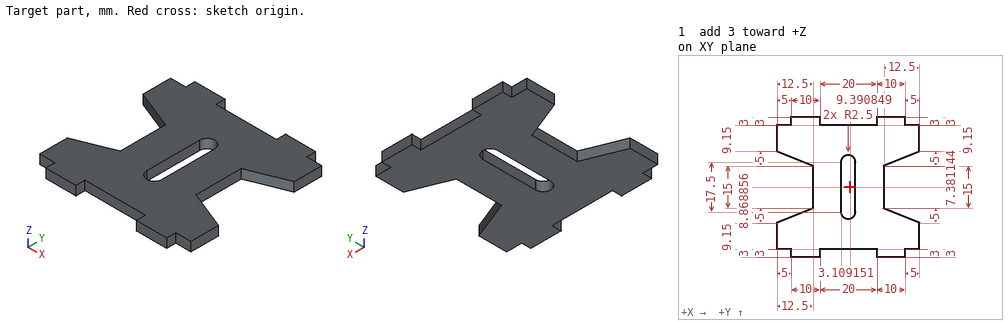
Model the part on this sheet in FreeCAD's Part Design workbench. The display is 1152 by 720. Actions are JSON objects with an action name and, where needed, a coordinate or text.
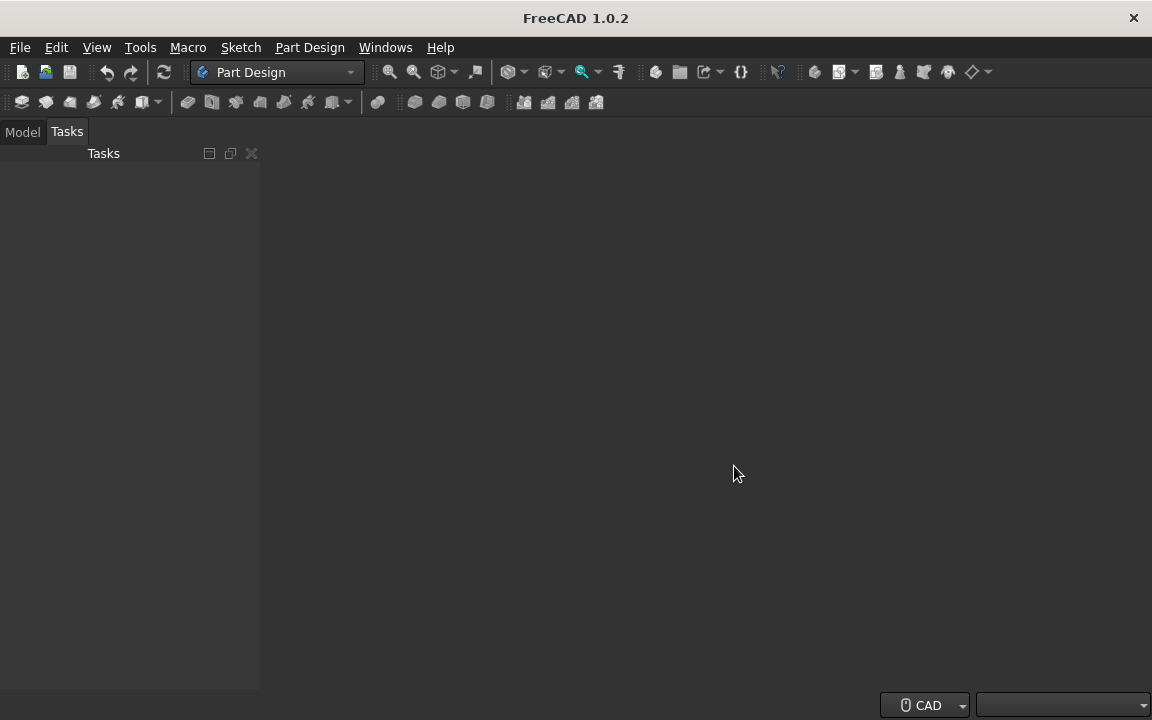
{"action": "left_click", "coordinate": [22, 72]}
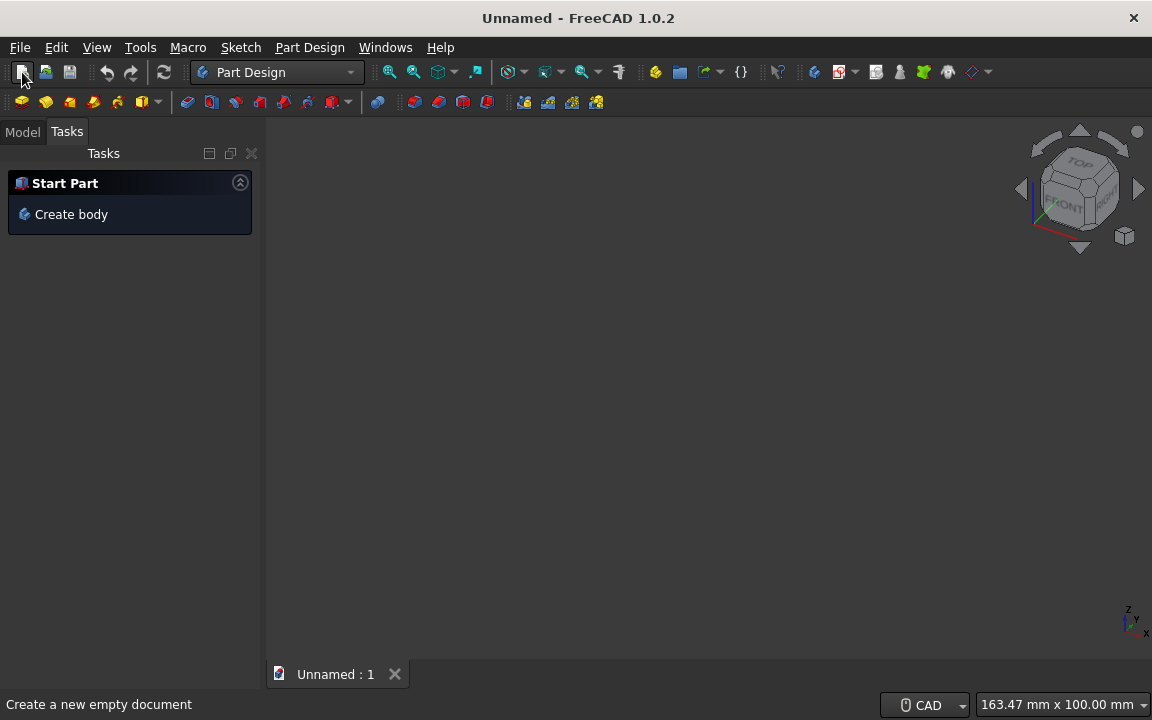
{"action": "left_click", "coordinate": [840, 72]}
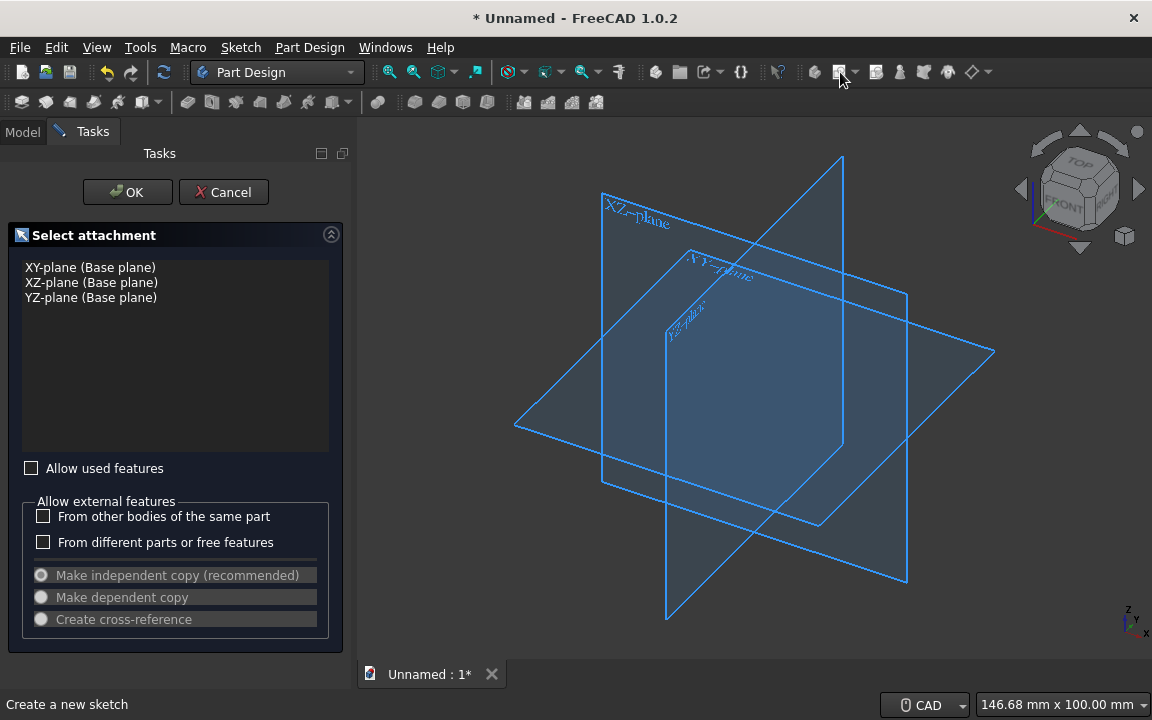
{"action": "left_click", "coordinate": [82, 268]}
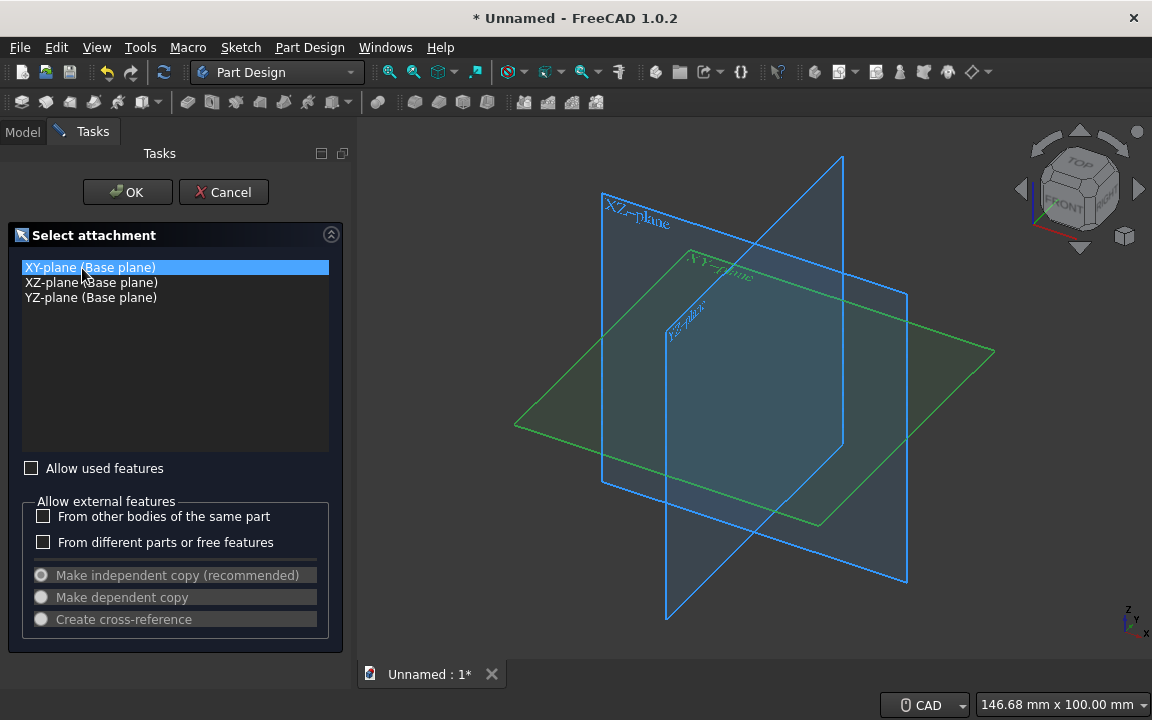
{"action": "left_click", "coordinate": [128, 192]}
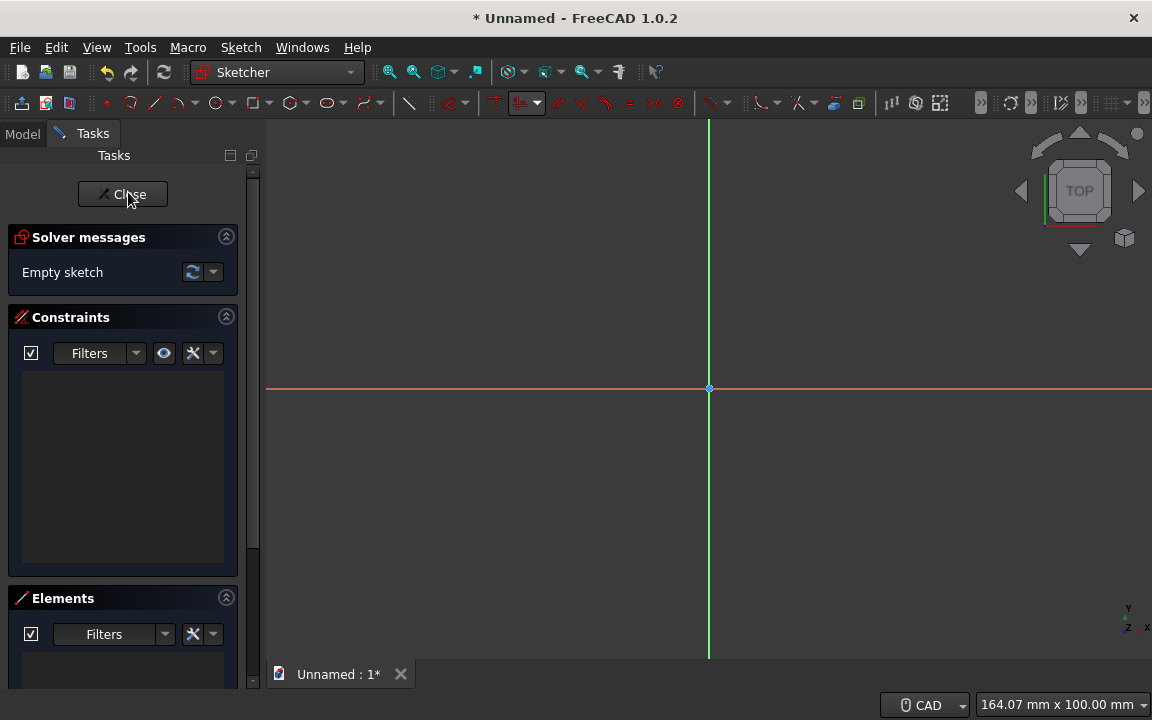
{"action": "left_click", "coordinate": [132, 104]}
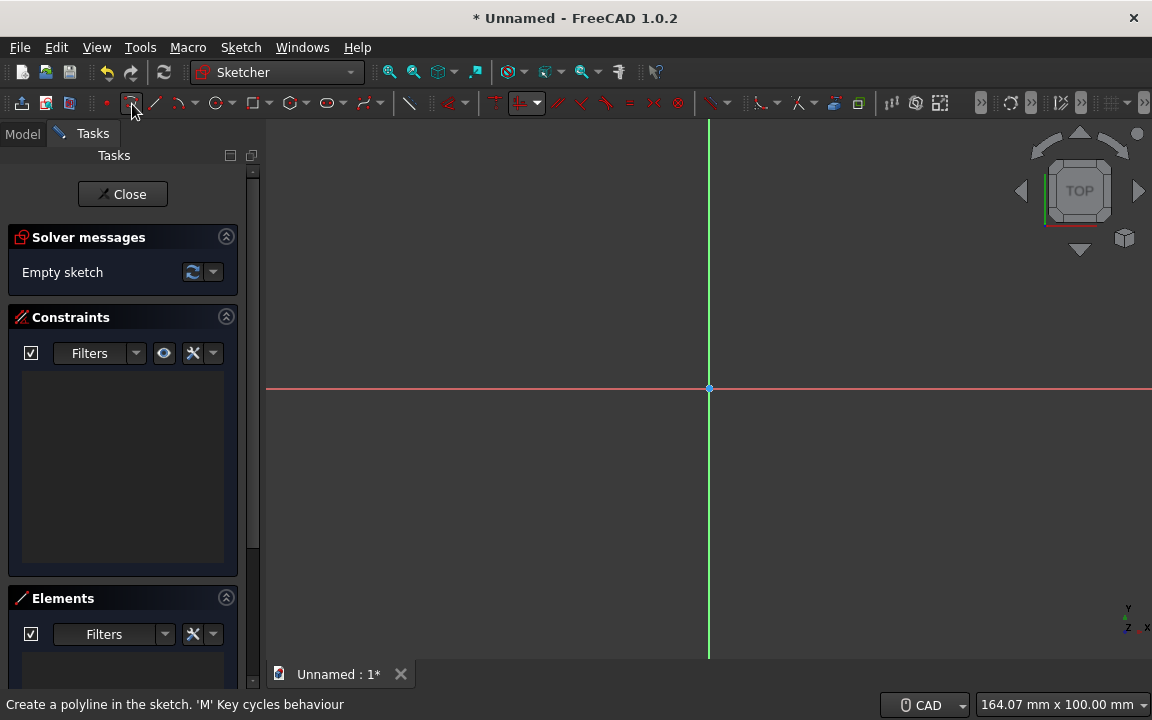
{"action": "left_click", "coordinate": [773, 349]}
{"action": "left_click", "coordinate": [841, 322]}
{"action": "left_click", "coordinate": [841, 273]}
{"action": "left_click", "coordinate": [814, 273]}
{"action": "left_click", "coordinate": [814, 257]}
{"action": "left_click", "coordinate": [760, 257]}
{"action": "left_click", "coordinate": [760, 273]}
{"action": "left_click", "coordinate": [652, 273]}
{"action": "left_click", "coordinate": [652, 257]}
{"action": "left_click", "coordinate": [598, 257]}
{"action": "left_click", "coordinate": [598, 273]}
{"action": "left_click", "coordinate": [571, 273]}
{"action": "left_click", "coordinate": [571, 322]}
{"action": "left_click", "coordinate": [638, 349]}
{"action": "left_click", "coordinate": [638, 430]}
{"action": "left_click", "coordinate": [571, 457]}
{"action": "left_click", "coordinate": [571, 507]}
{"action": "left_click", "coordinate": [598, 507]}
{"action": "left_click", "coordinate": [598, 523]}
{"action": "left_click", "coordinate": [652, 523]}
{"action": "left_click", "coordinate": [652, 507]}
{"action": "left_click", "coordinate": [760, 507]}
{"action": "left_click", "coordinate": [760, 523]}
{"action": "left_click", "coordinate": [814, 523]}
{"action": "left_click", "coordinate": [814, 507]}
{"action": "left_click", "coordinate": [841, 507]}
{"action": "left_click", "coordinate": [841, 457]}
{"action": "left_click", "coordinate": [773, 430]}
{"action": "left_click", "coordinate": [773, 350]}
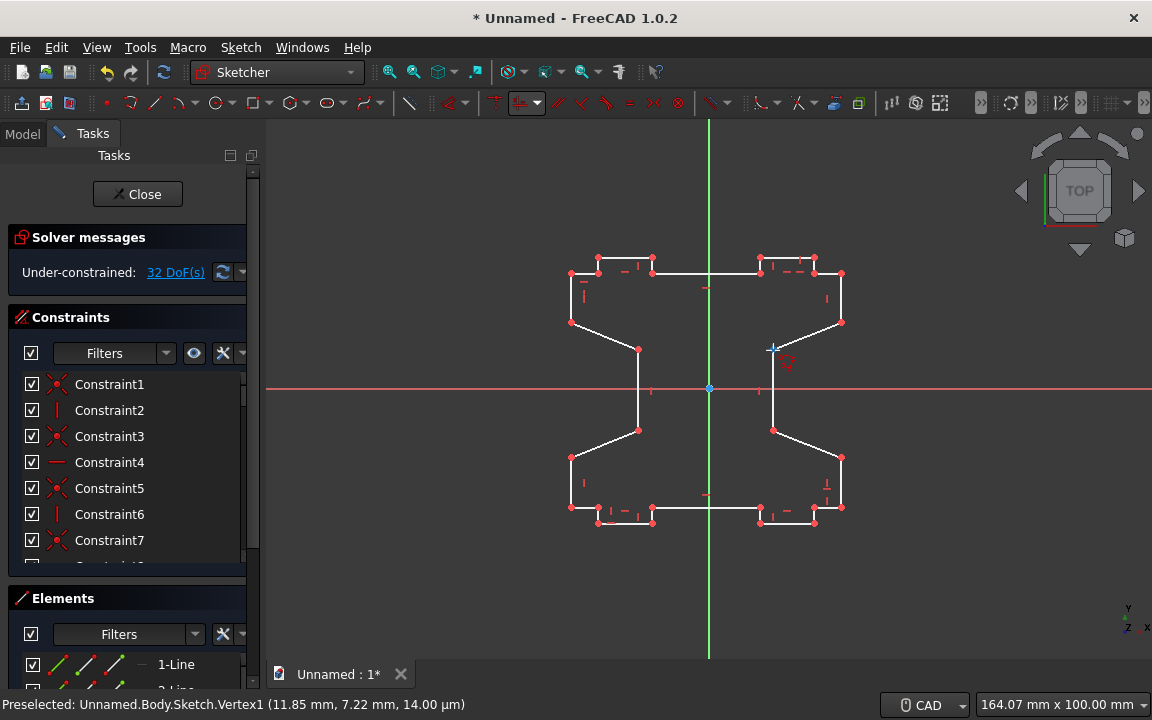
{"action": "left_click", "coordinate": [328, 104]}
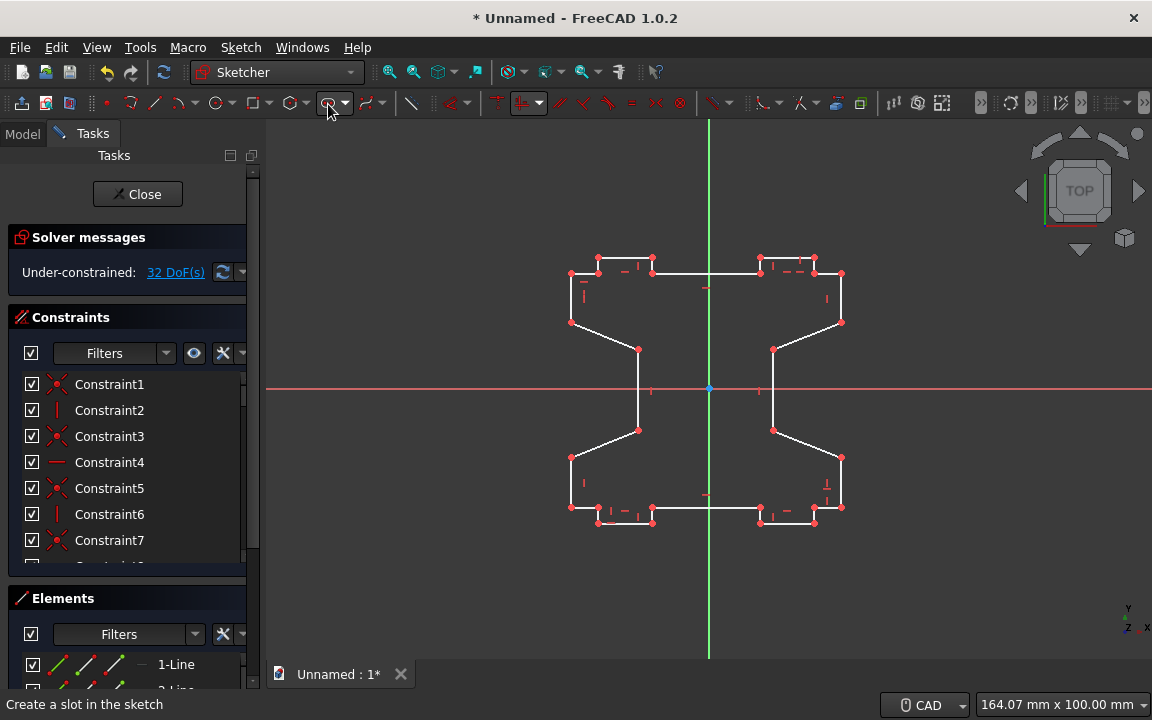
{"action": "scroll", "coordinate": [706, 437], "scroll_direction": "up", "scroll_amount": 8}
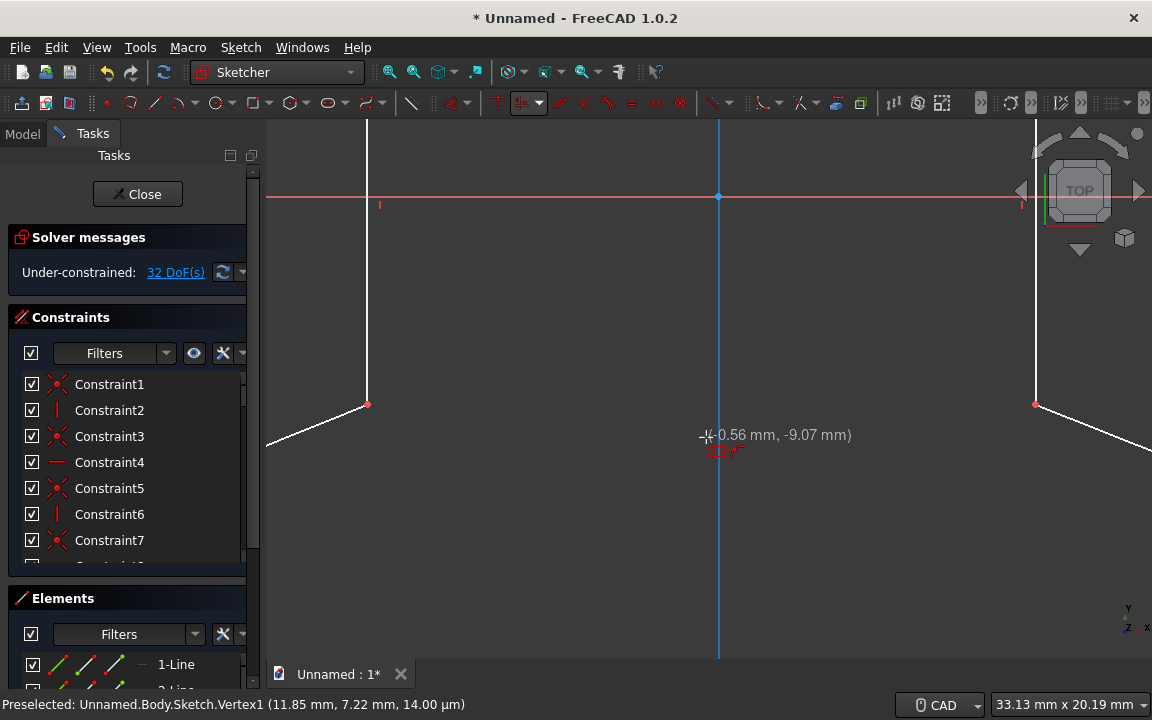
{"action": "left_click", "coordinate": [703, 434]}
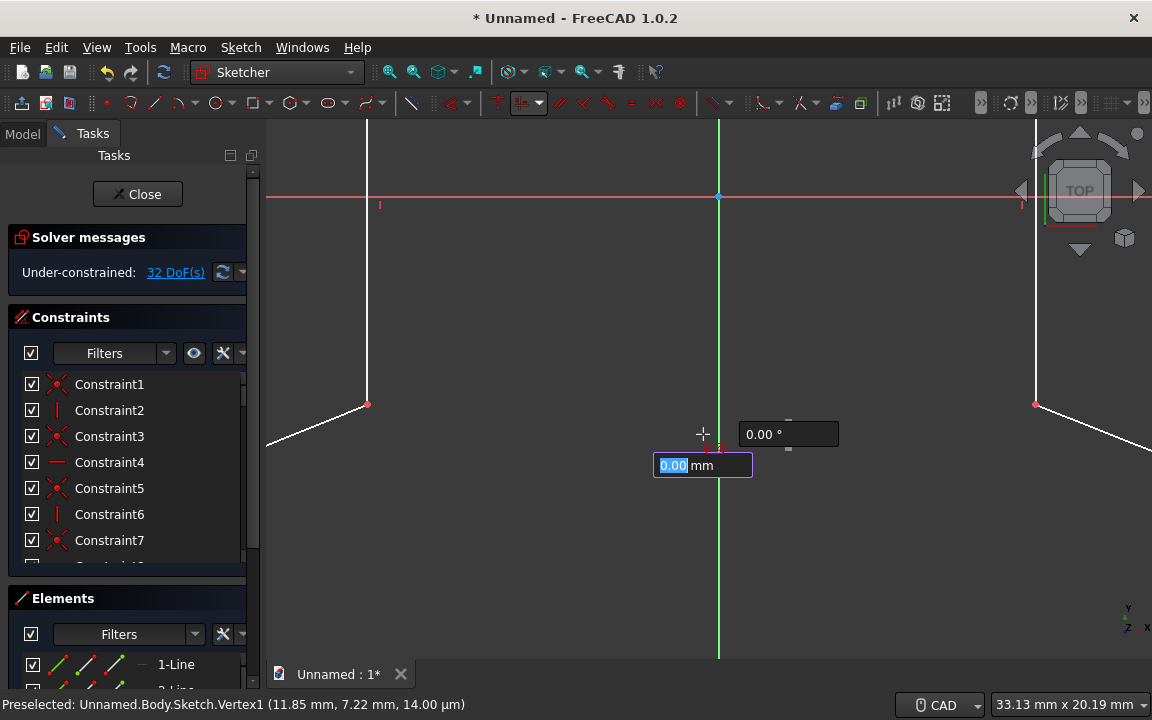
{"action": "scroll", "coordinate": [620, 451], "scroll_direction": "down", "scroll_amount": 7}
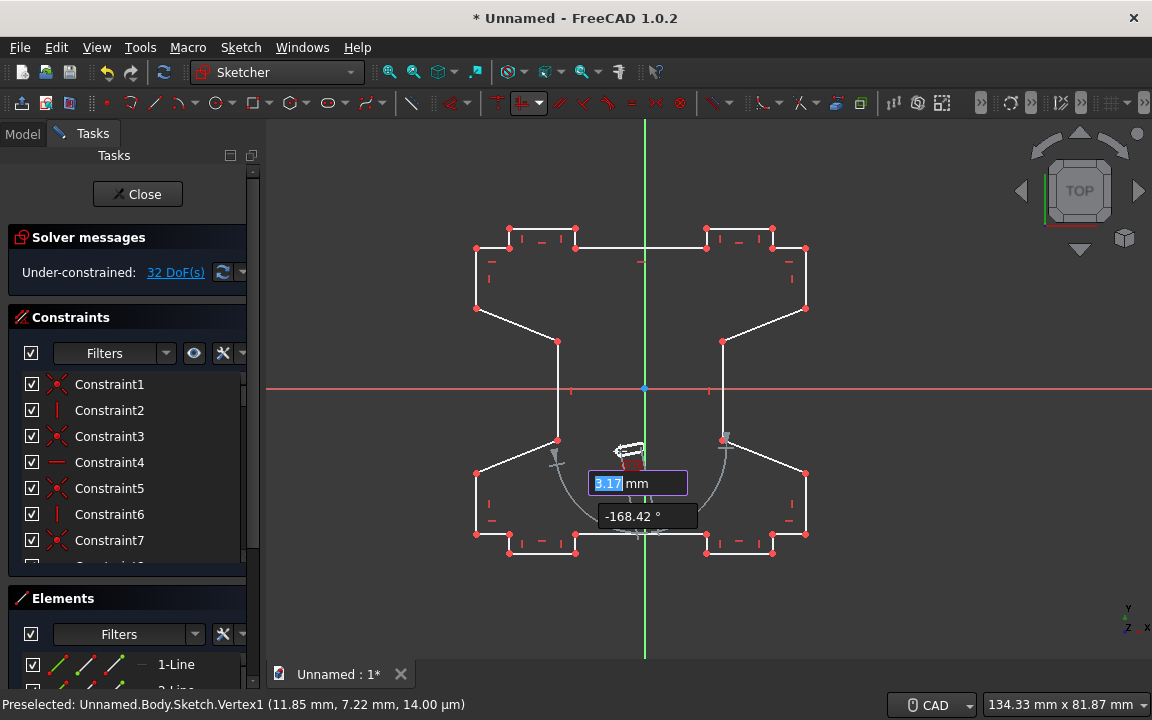
{"action": "scroll", "coordinate": [641, 332], "scroll_direction": "up", "scroll_amount": 7}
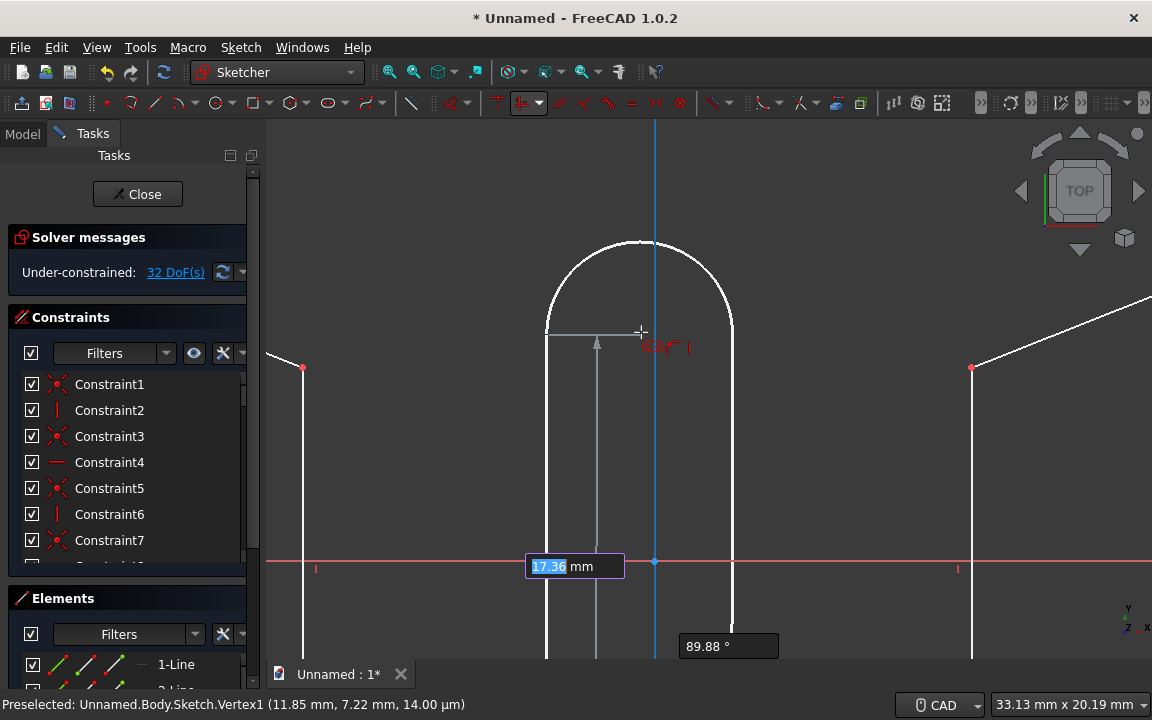
{"action": "left_click", "coordinate": [639, 330]}